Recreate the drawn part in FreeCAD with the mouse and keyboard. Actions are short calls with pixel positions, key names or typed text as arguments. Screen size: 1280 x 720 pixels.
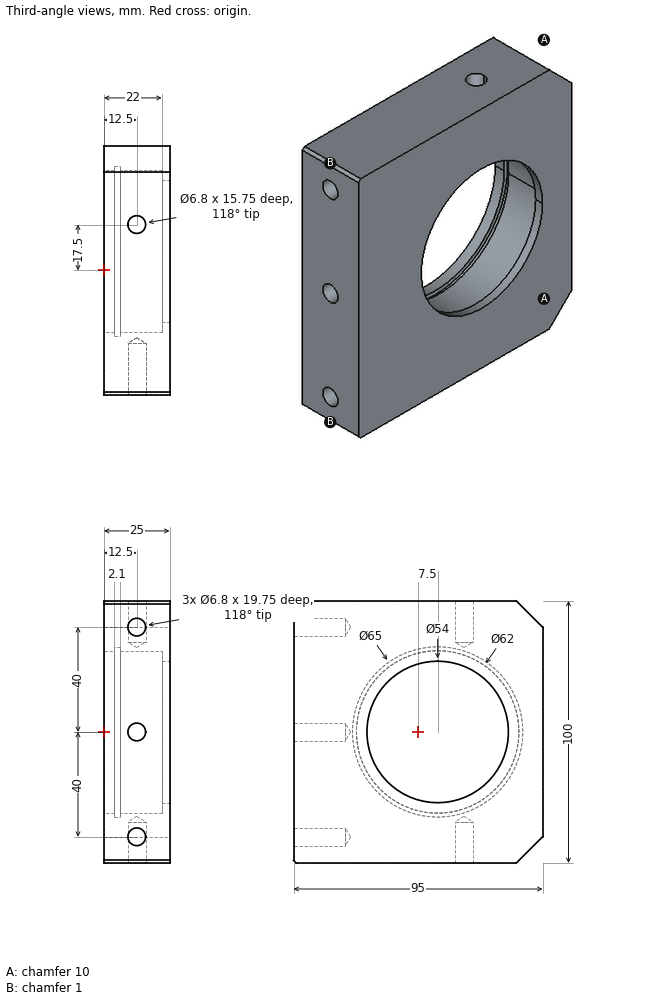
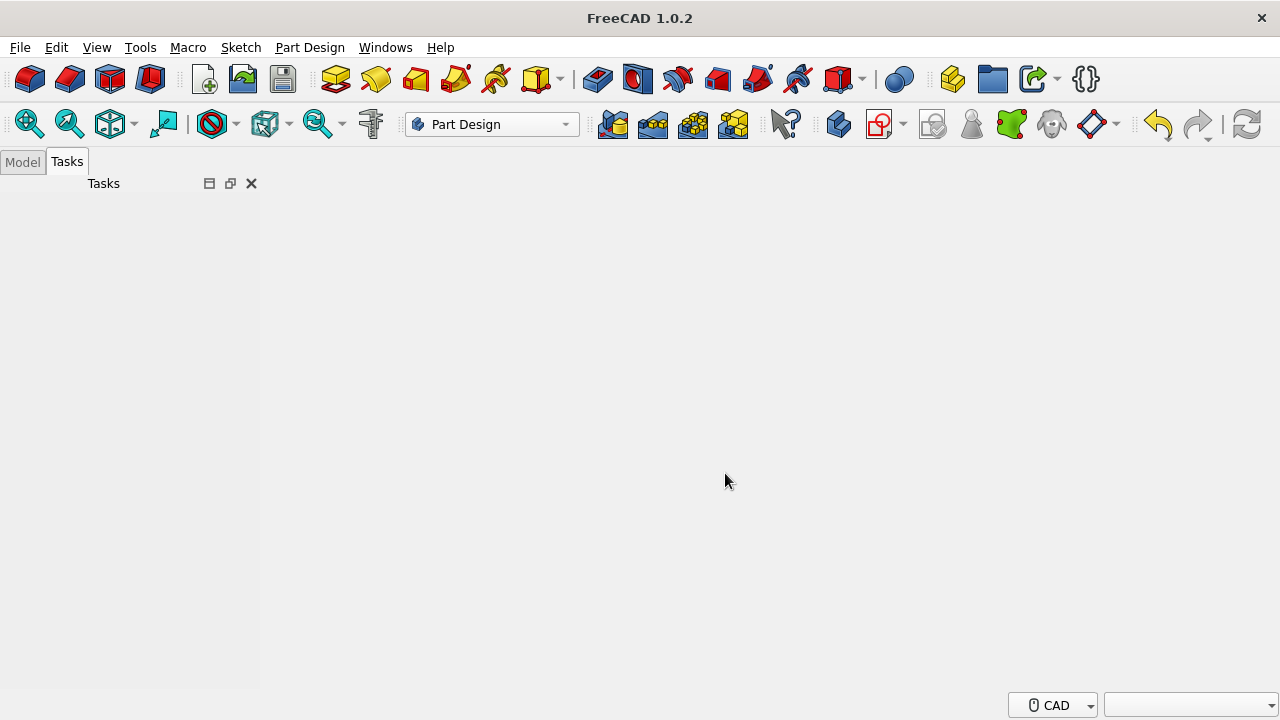
key(ctrl+n)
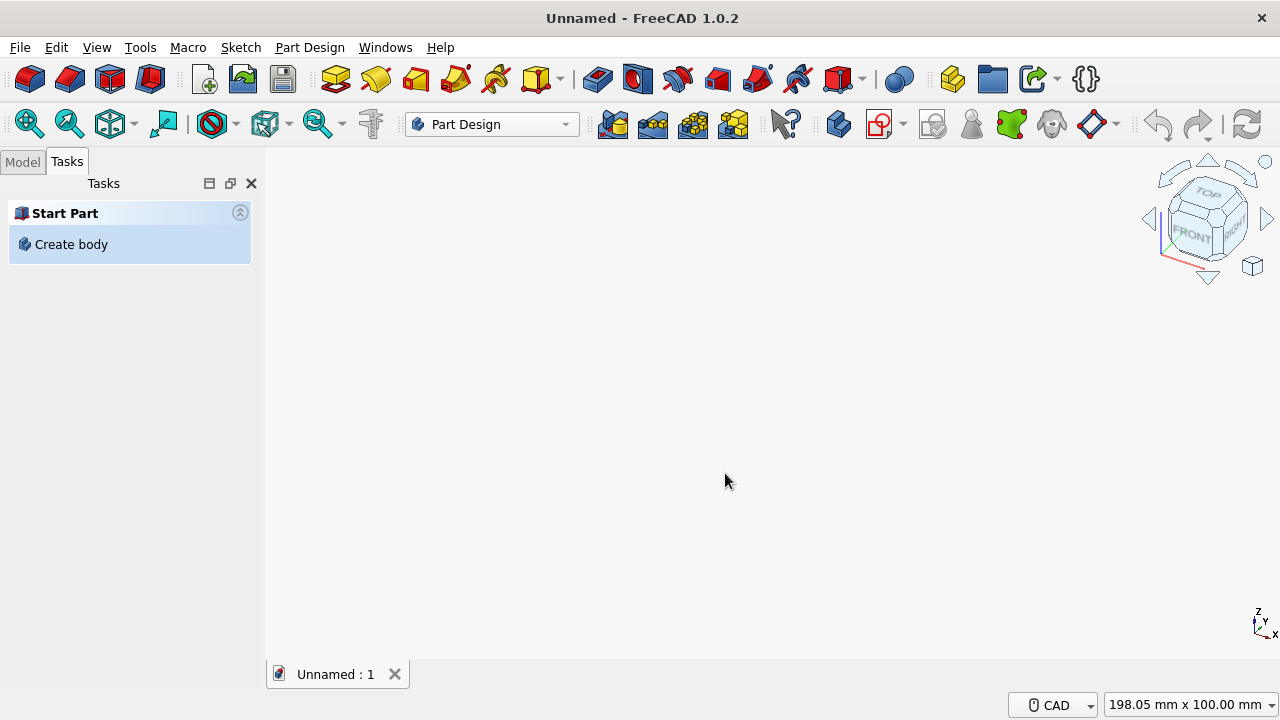
click(880, 124)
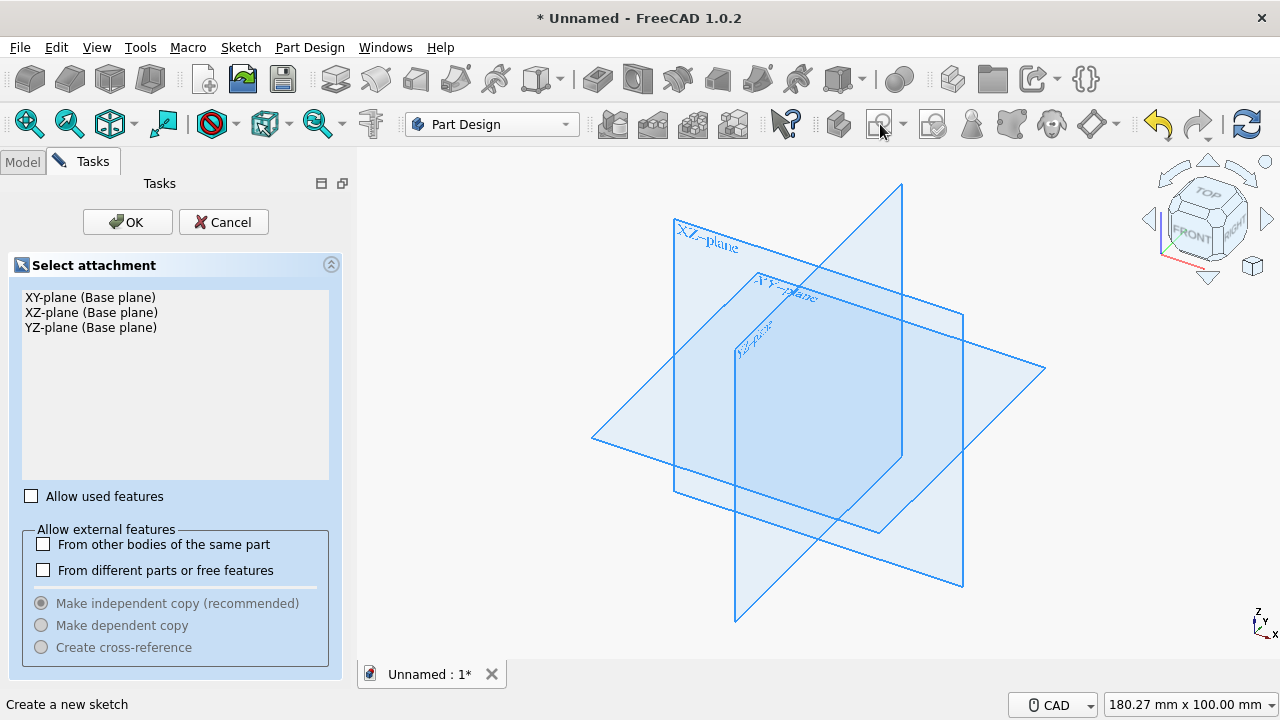
click(82, 328)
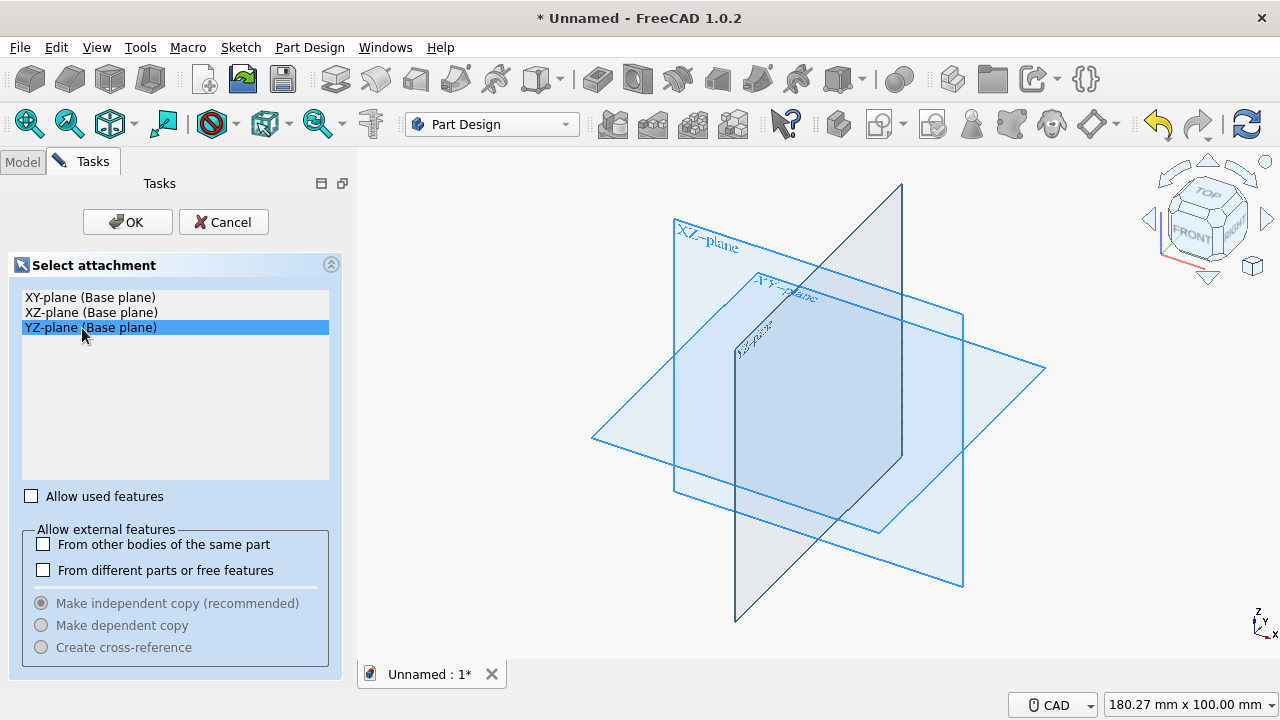
click(128, 222)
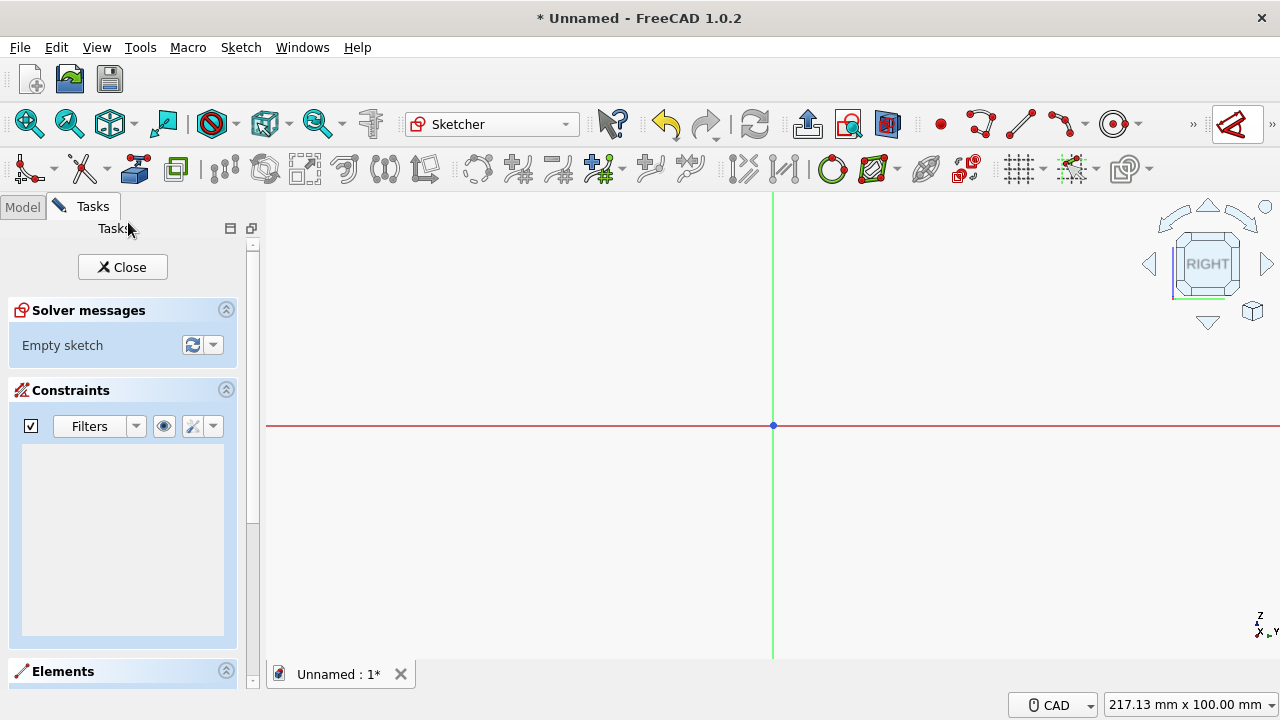
scroll(565, 425, down, 2)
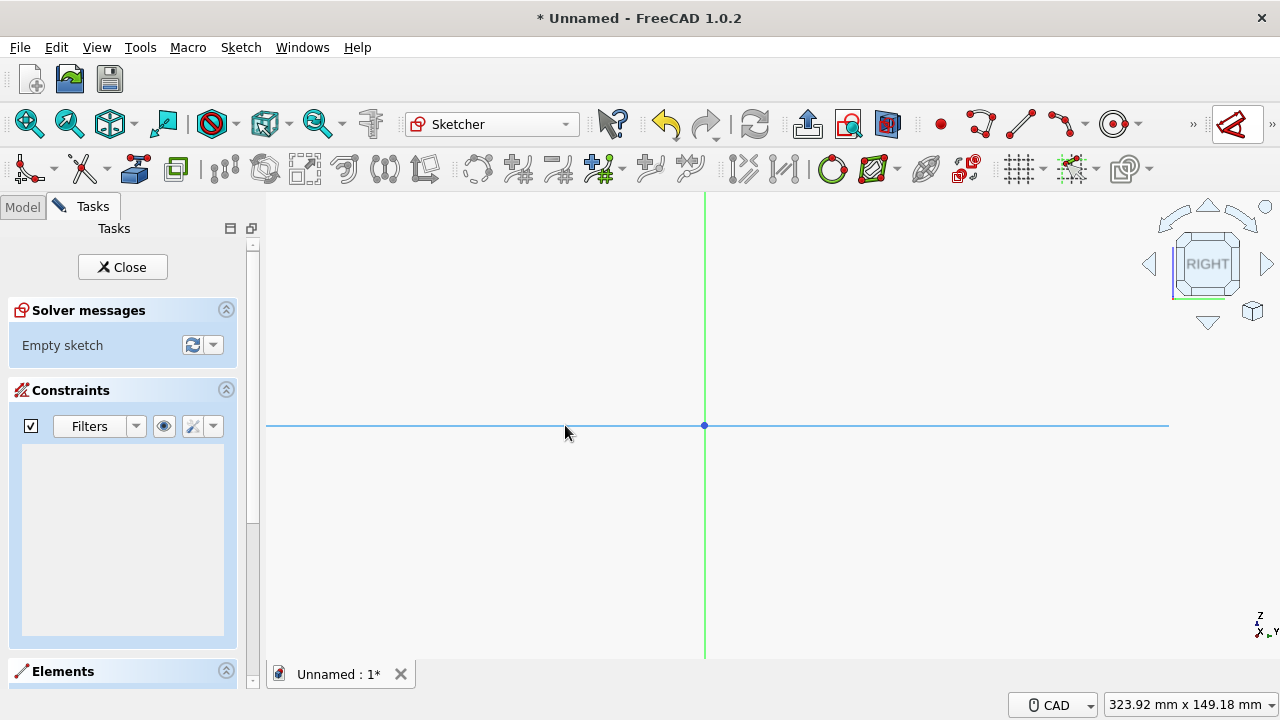
key(g)
key(v)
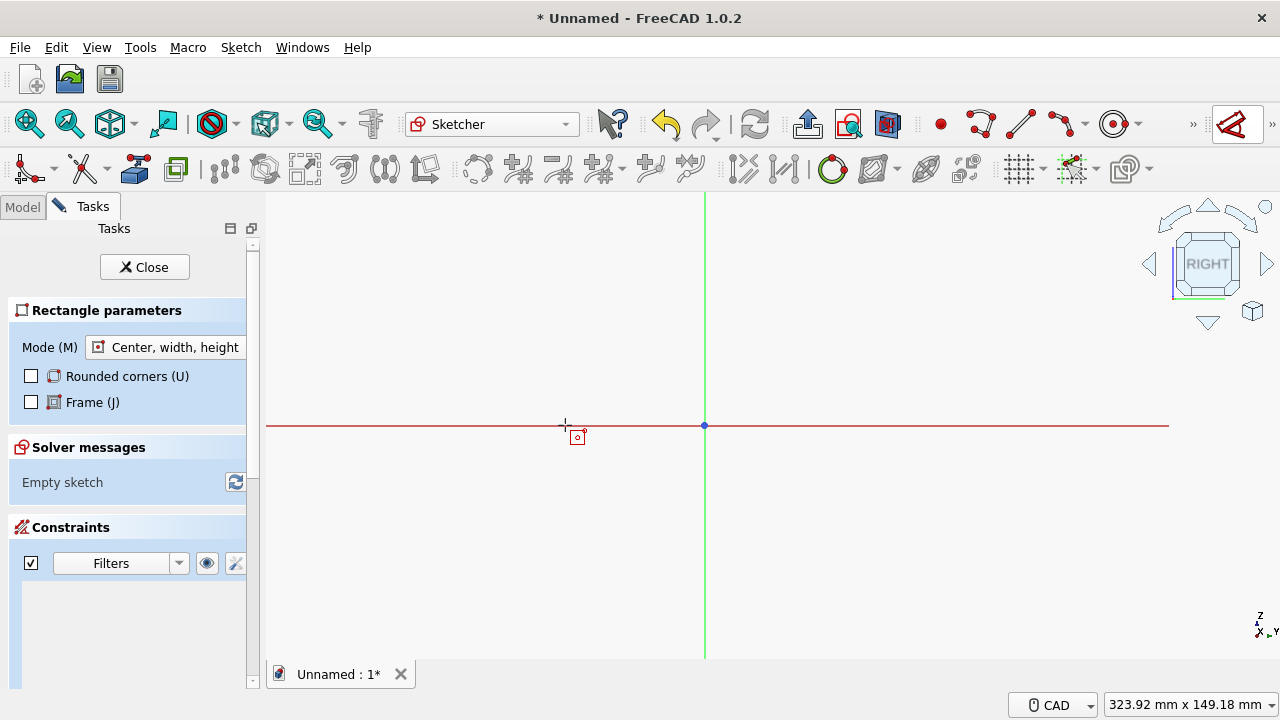
click(705, 426)
click(853, 269)
key(Escape)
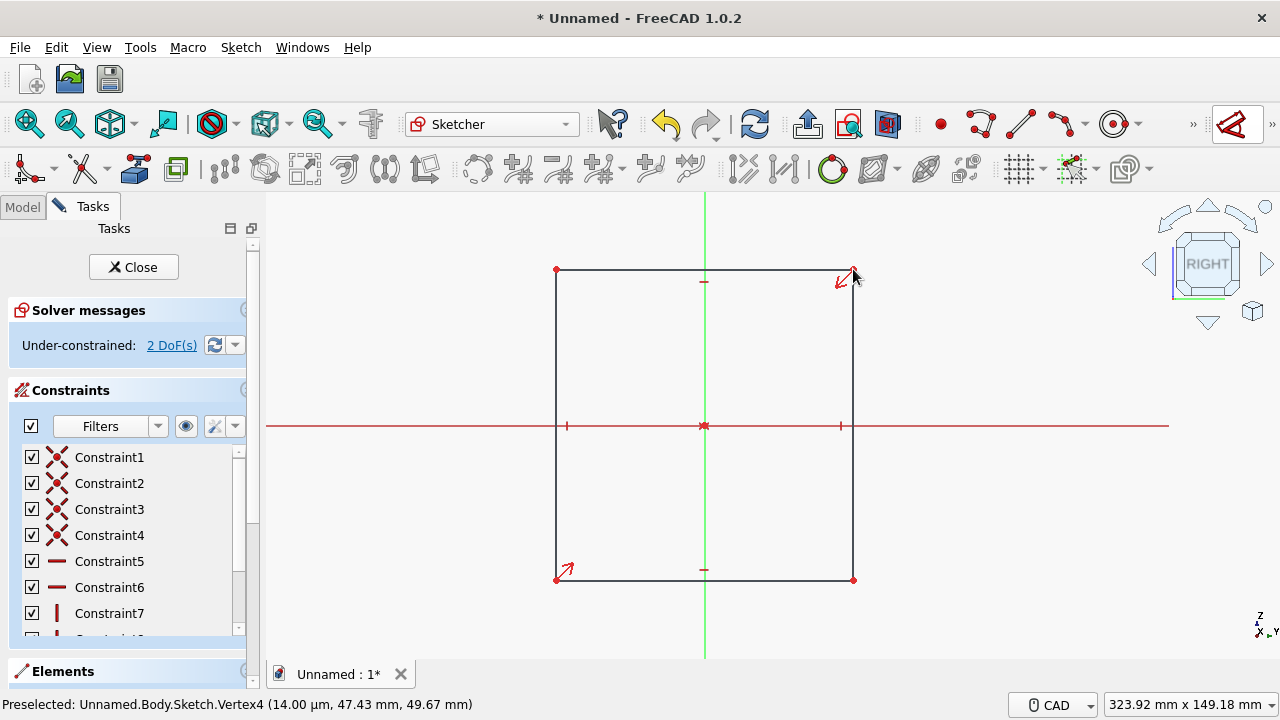
click(1232, 124)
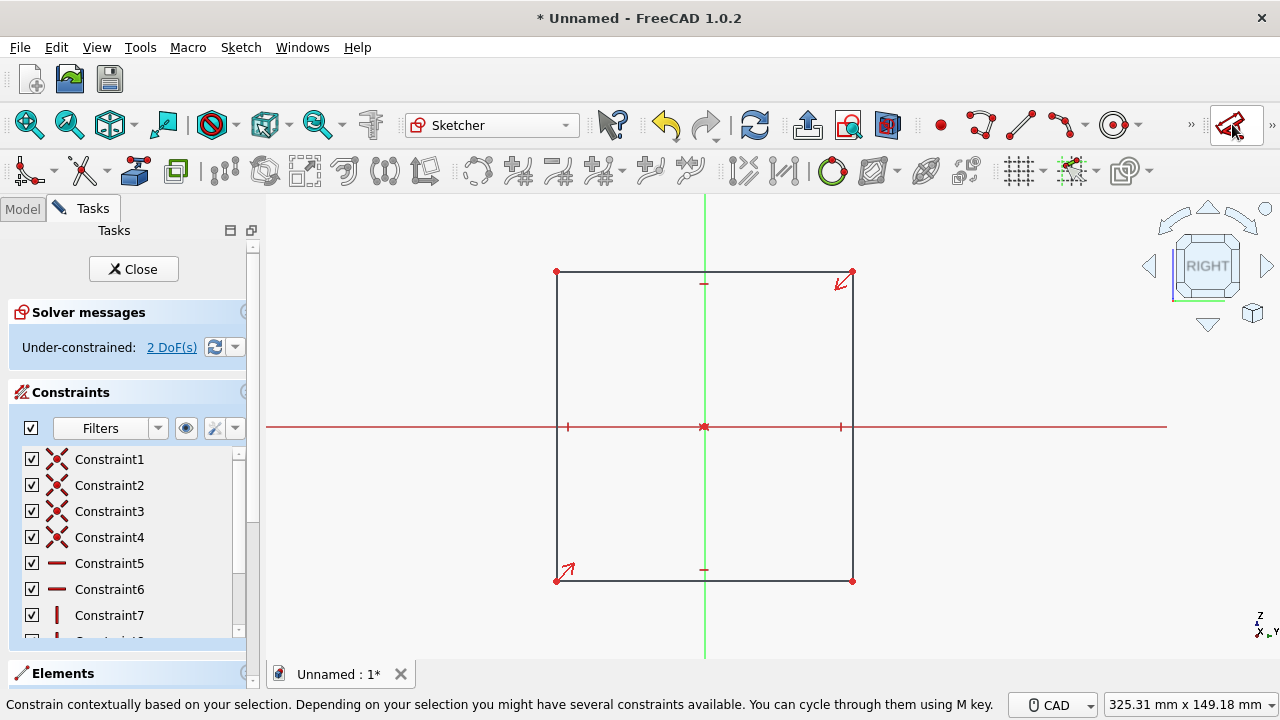
click(646, 581)
click(637, 615)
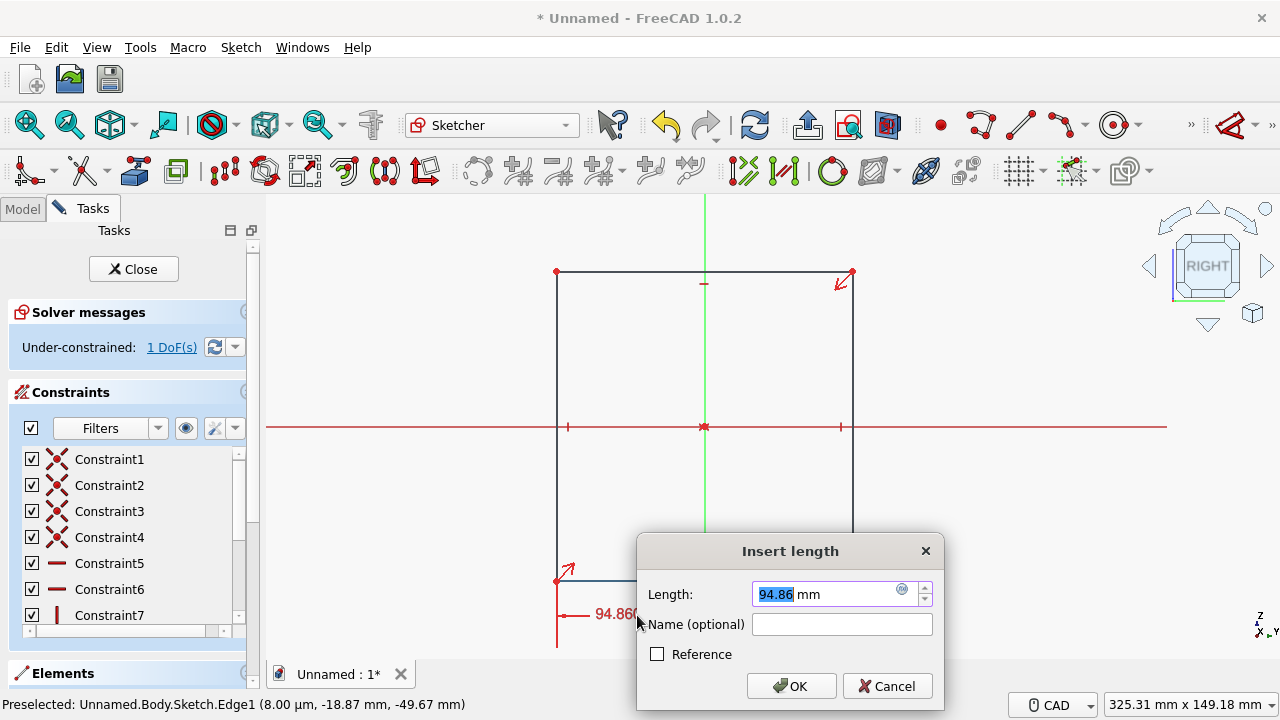
text(95)
key(Return)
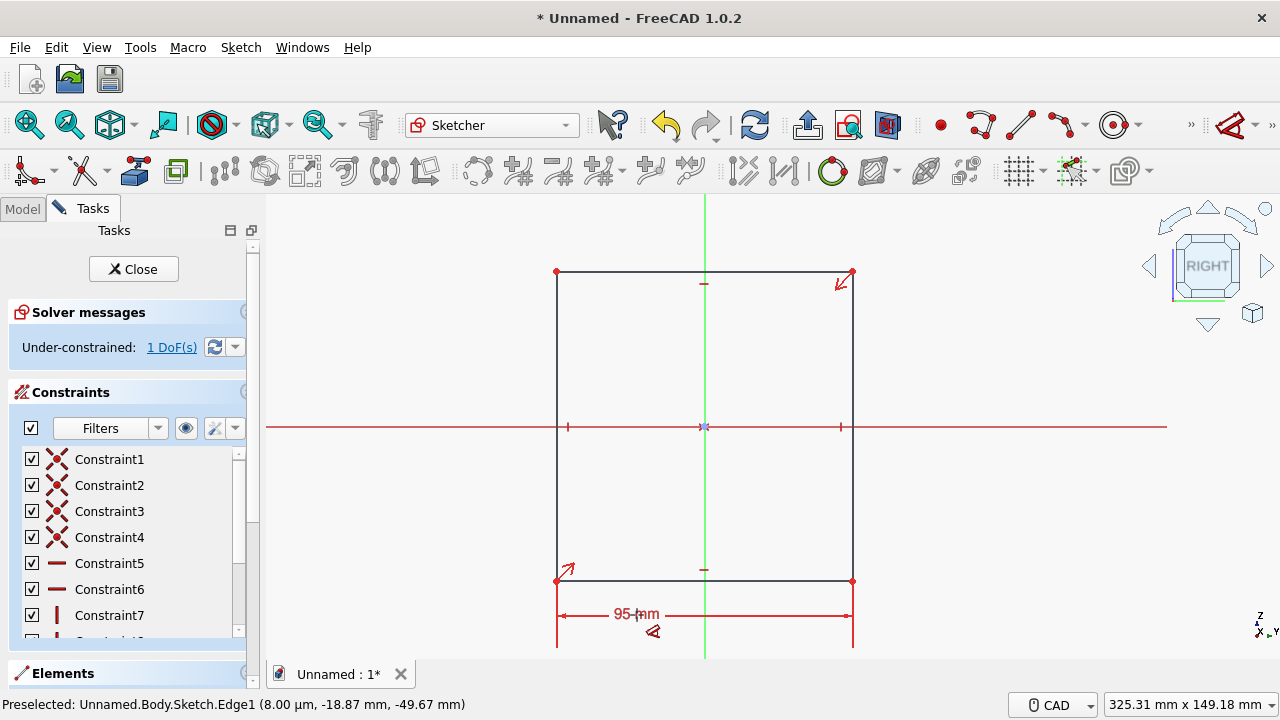
click(853, 488)
click(887, 355)